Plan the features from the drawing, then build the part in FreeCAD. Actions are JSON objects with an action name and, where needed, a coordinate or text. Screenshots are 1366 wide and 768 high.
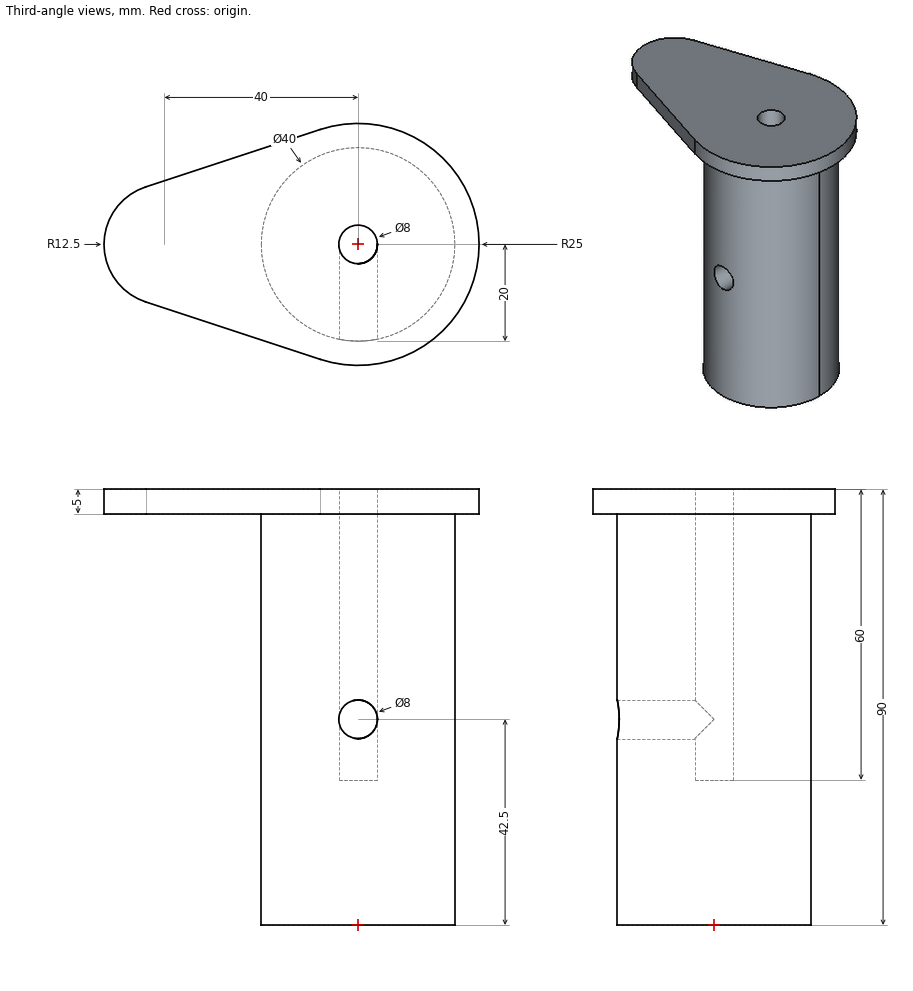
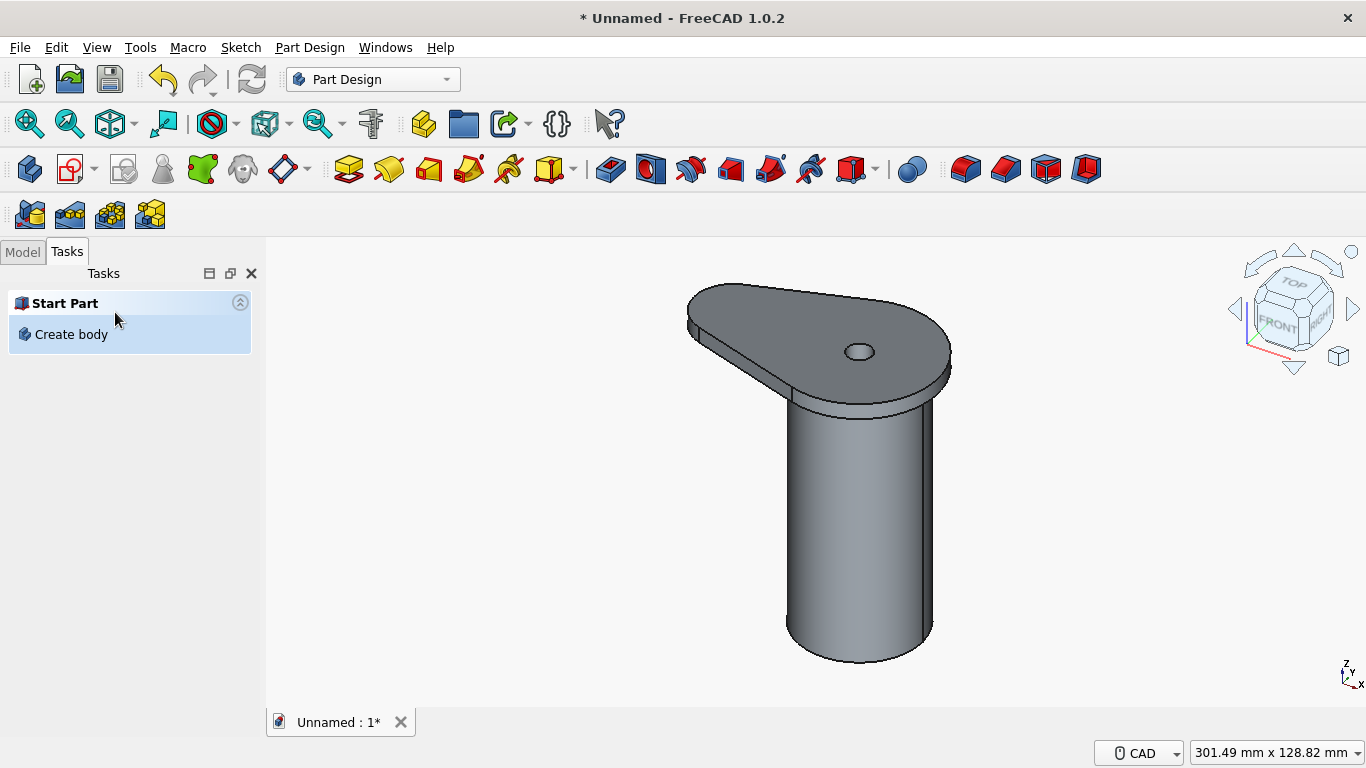
{"action": "left_click", "coordinate": [70, 170]}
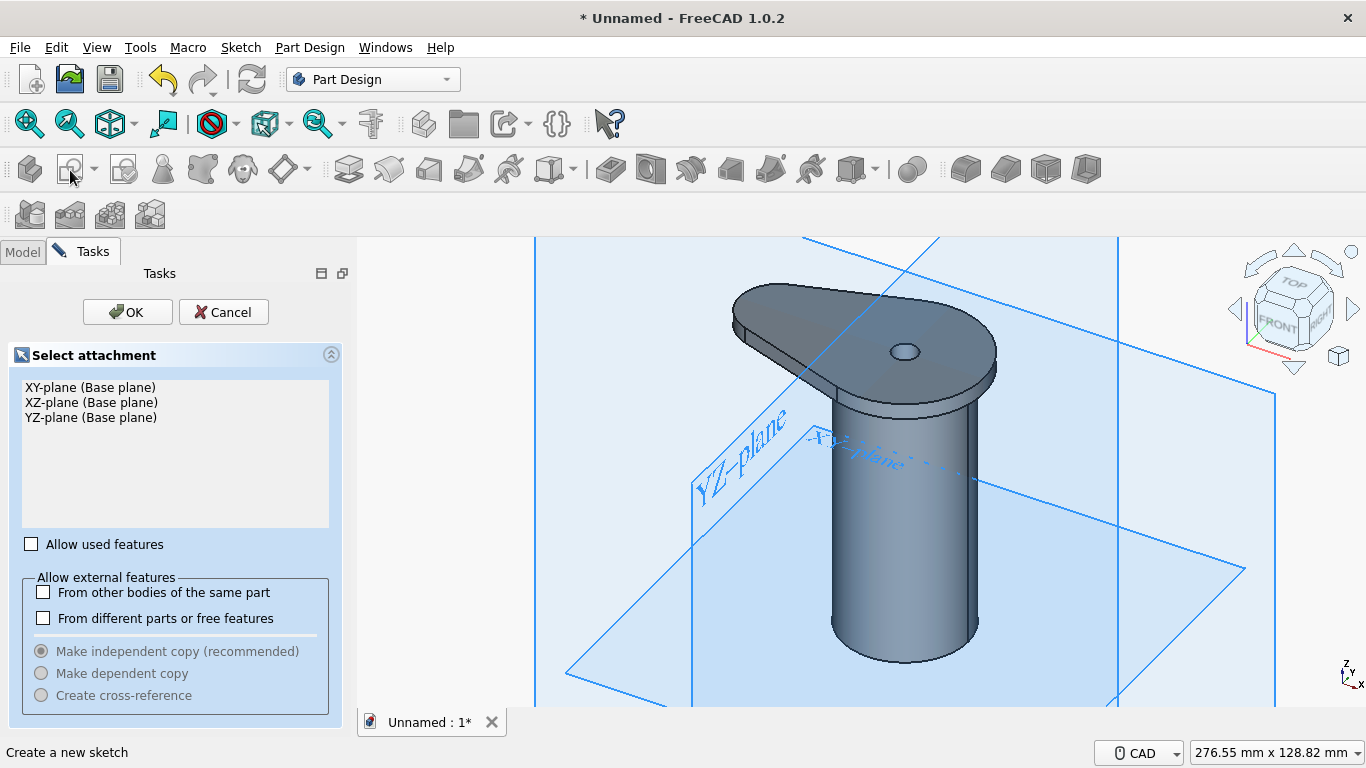
{"action": "left_click", "coordinate": [82, 402]}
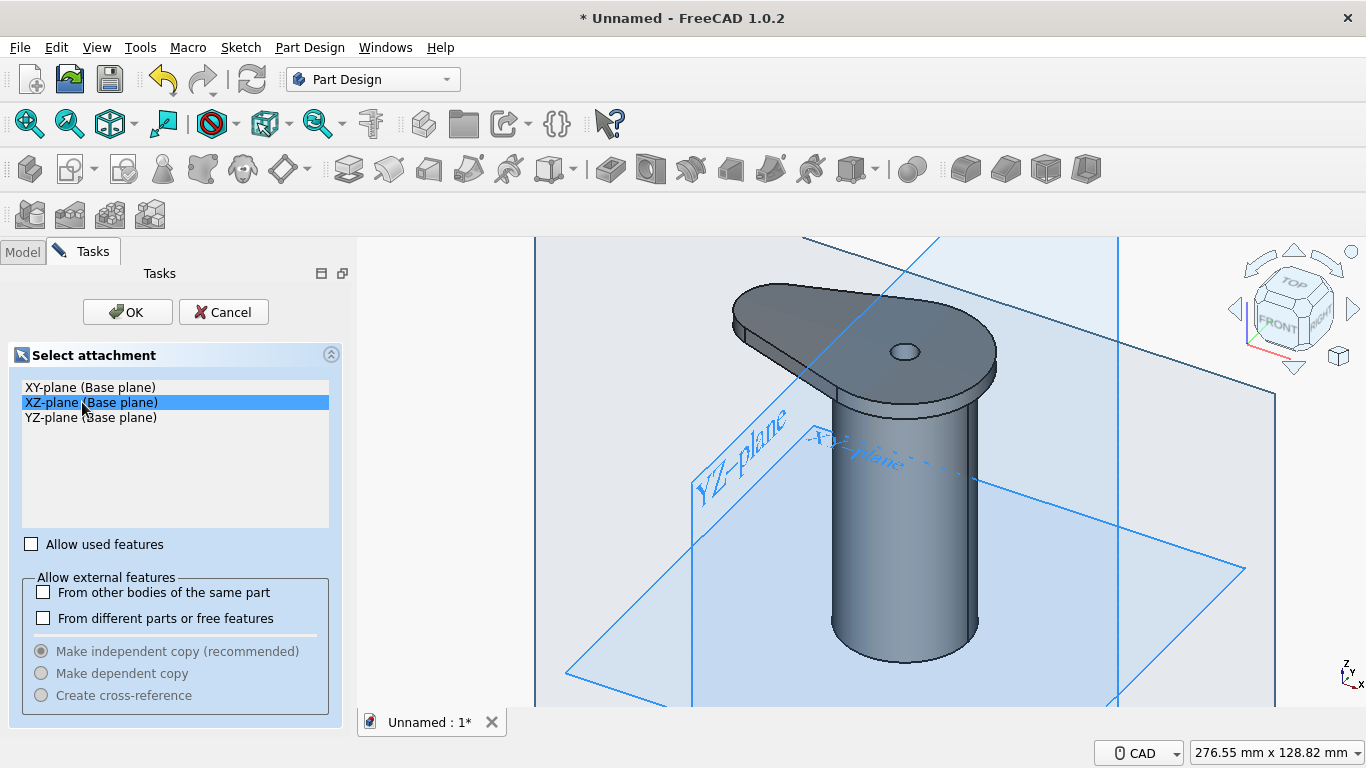
{"action": "left_click", "coordinate": [128, 312]}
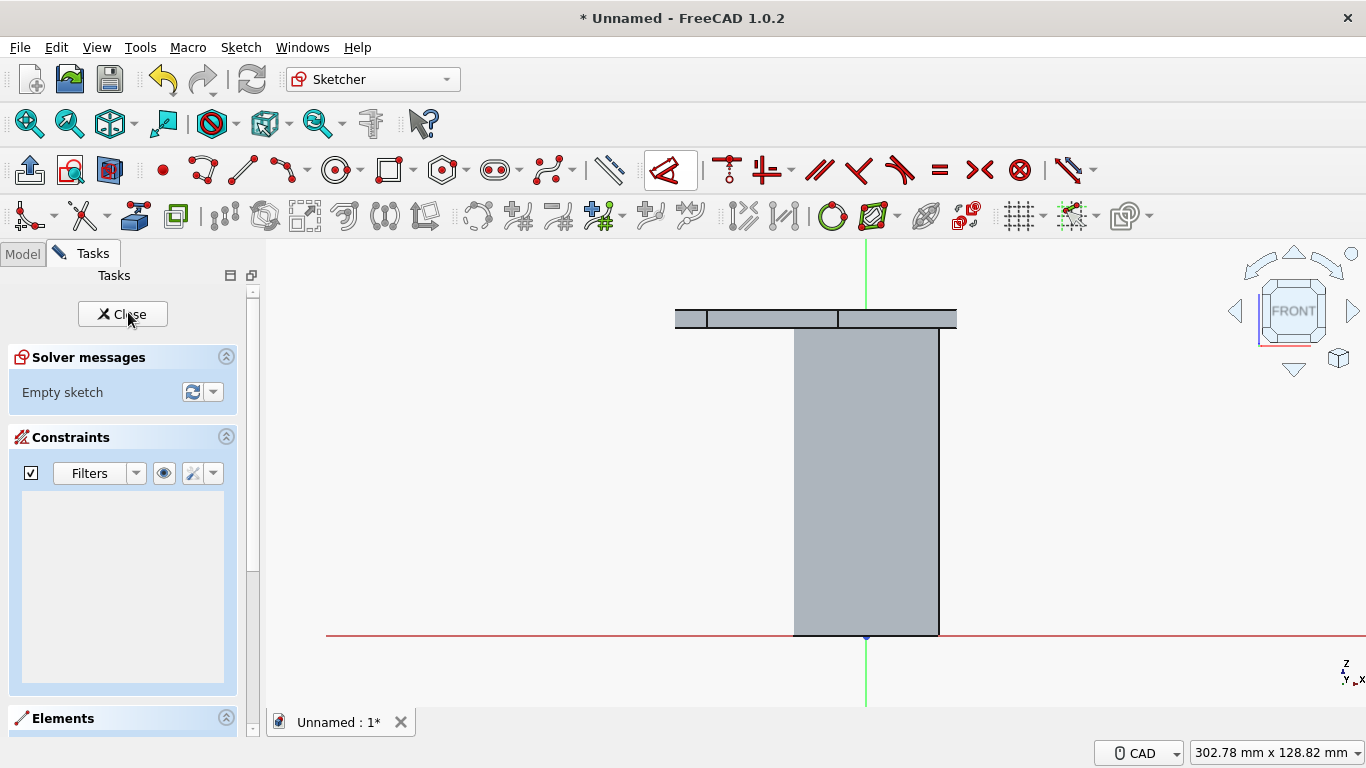
{"action": "left_click", "coordinate": [110, 170]}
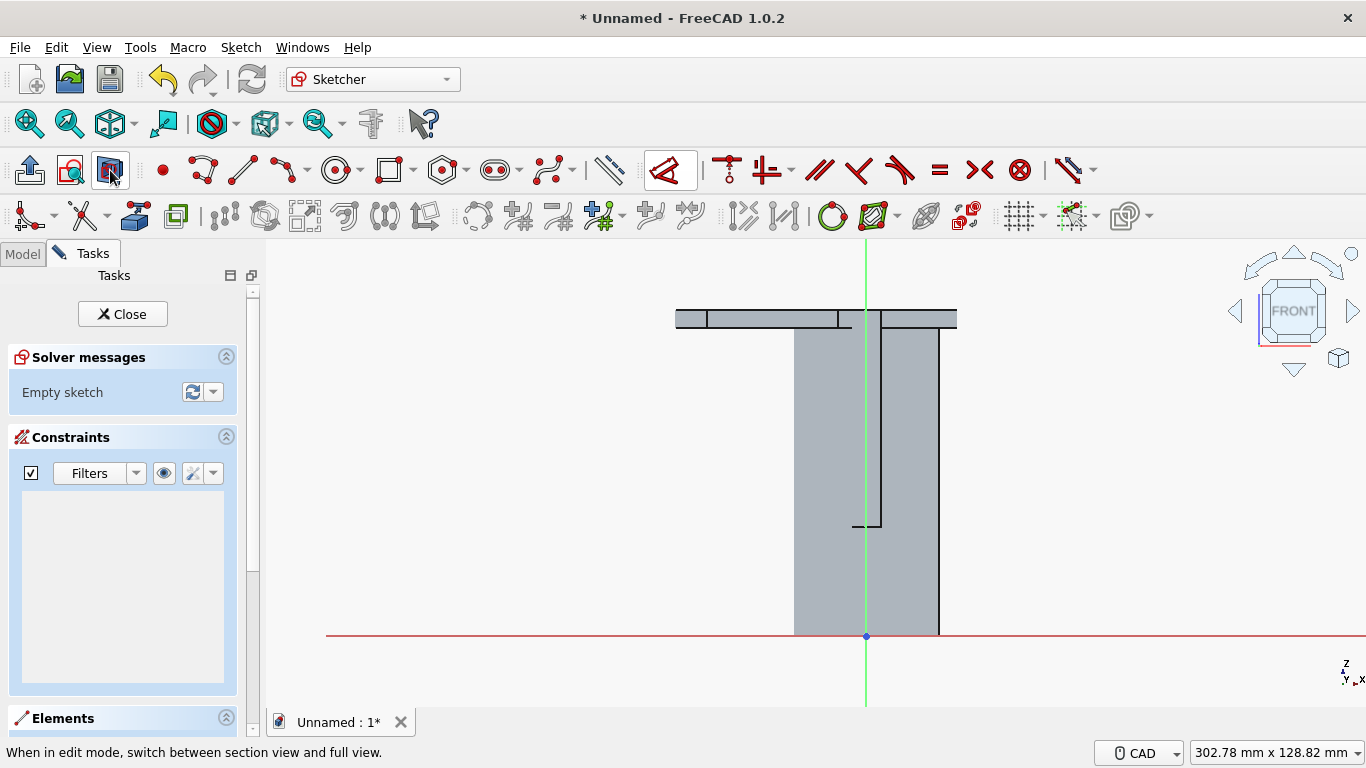
{"action": "scroll", "coordinate": [878, 483], "scroll_direction": "up", "scroll_amount": 12}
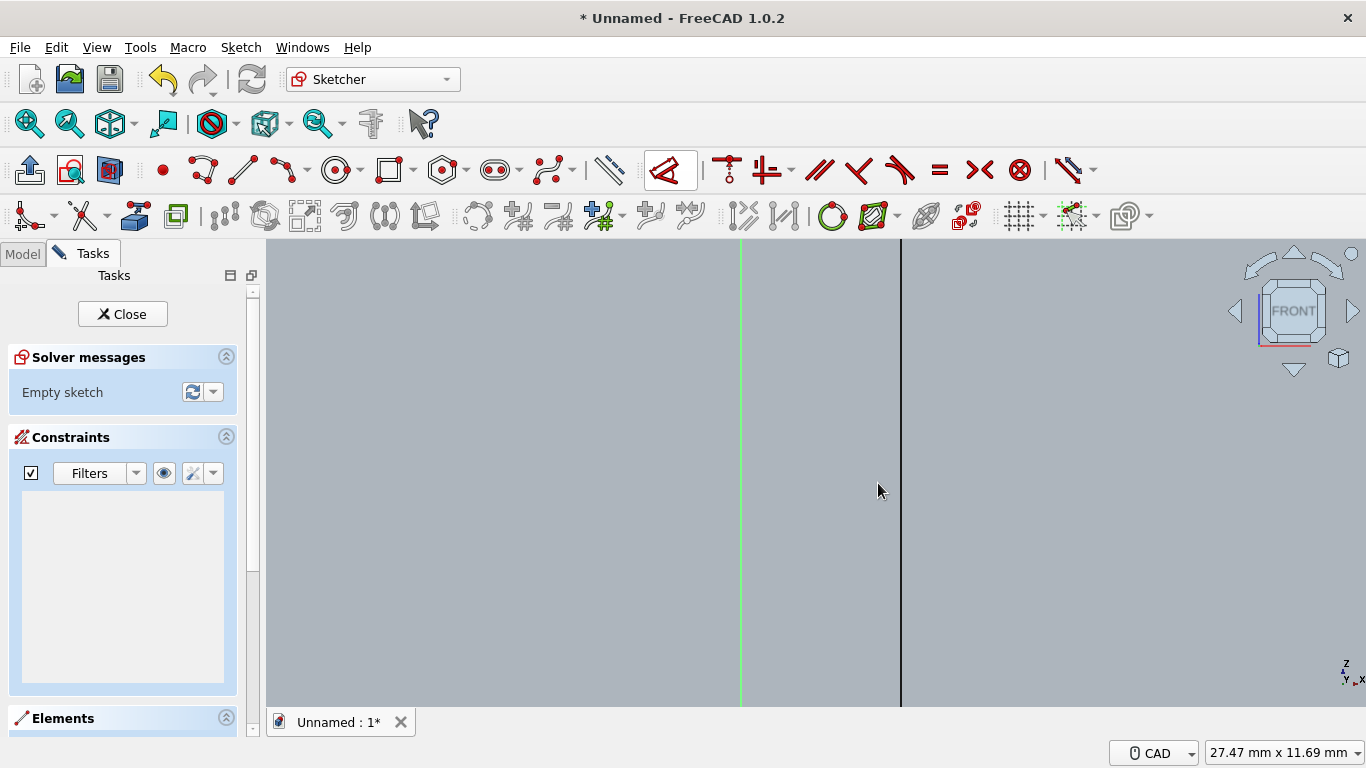
{"action": "key", "text": "g c"}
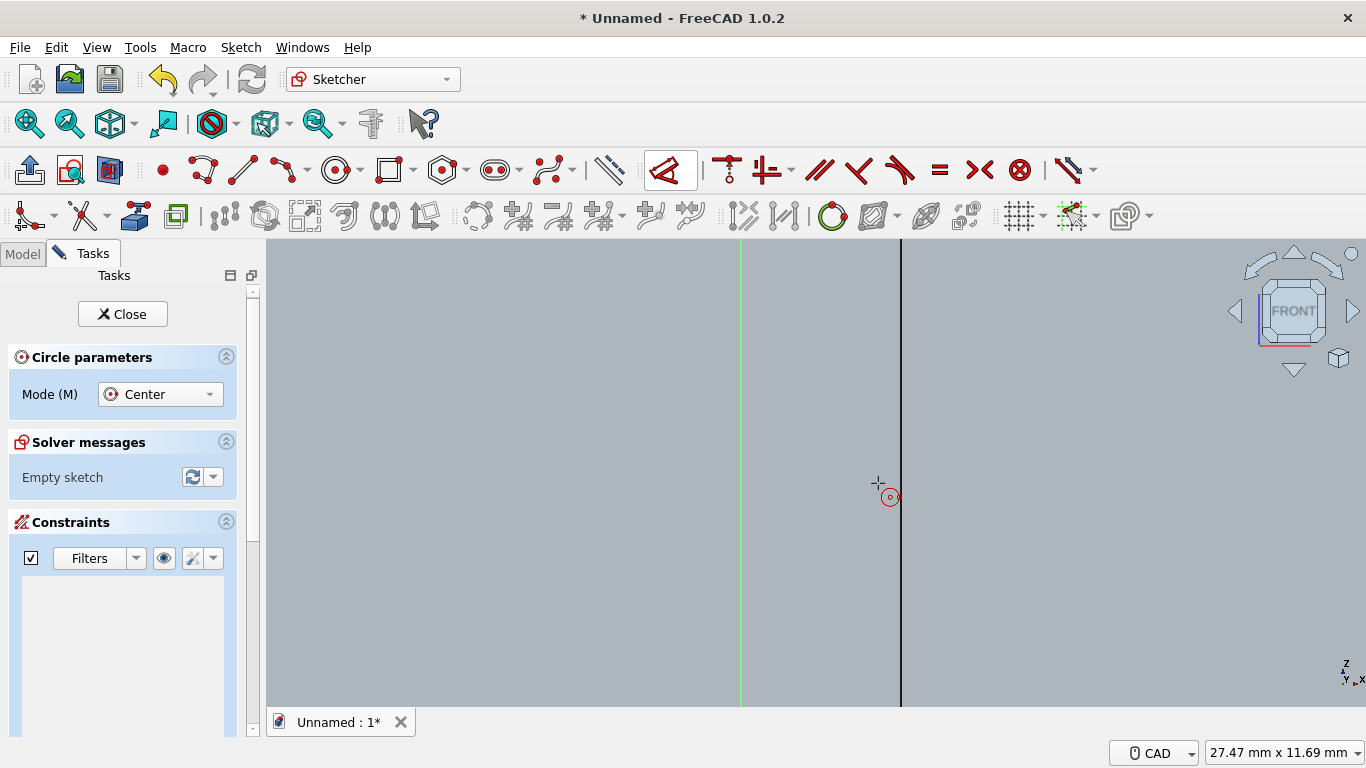
{"action": "left_click", "coordinate": [741, 468]}
{"action": "mouse_move", "coordinate": [854, 354]}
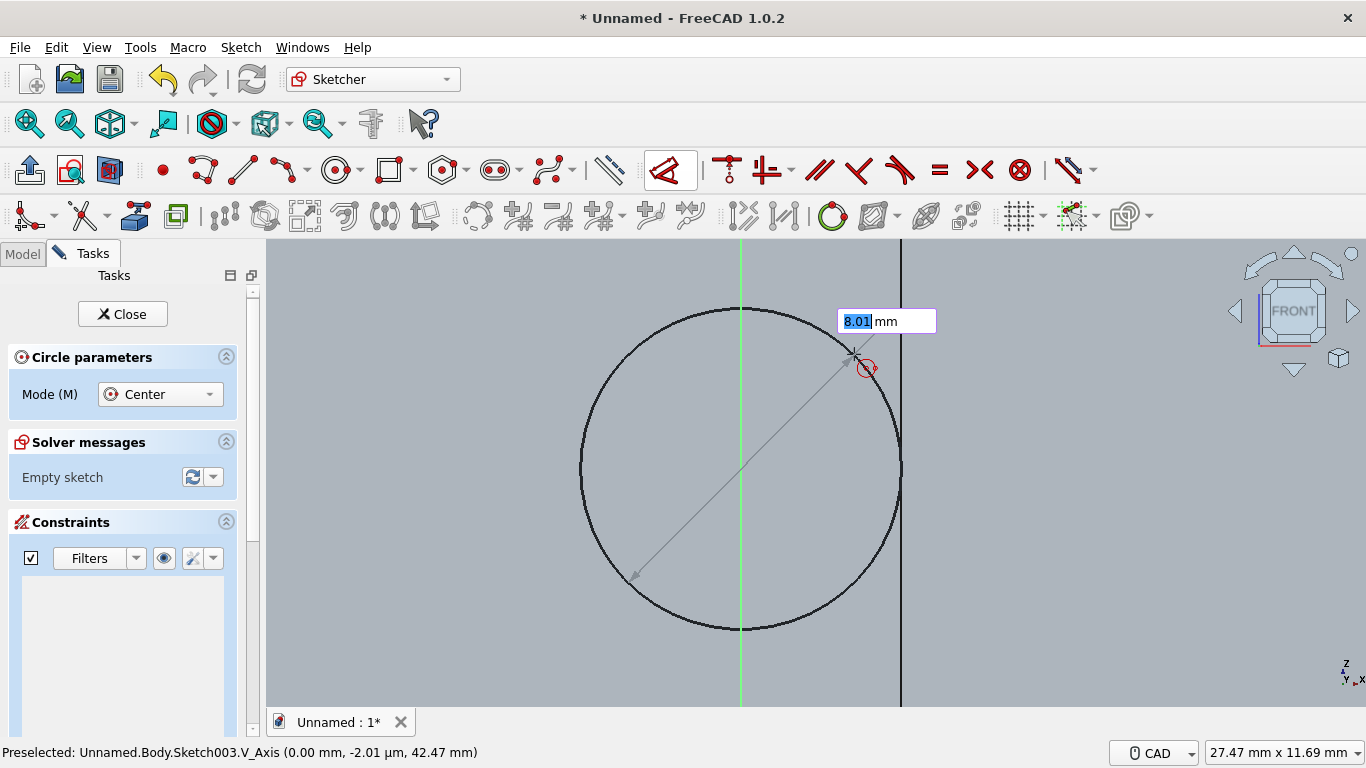
{"action": "type", "text": "8"}
{"action": "key", "text": "Return"}
{"action": "key", "text": "Escape"}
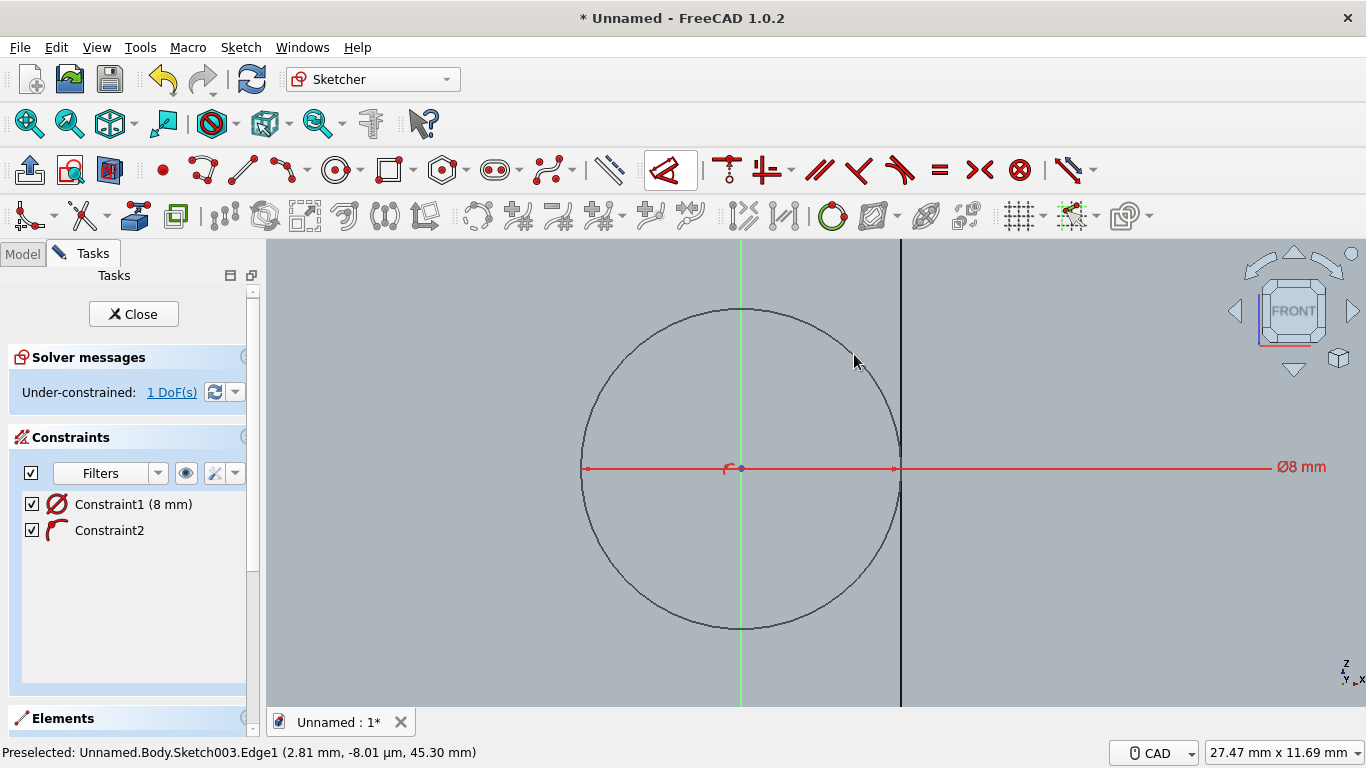
{"action": "left_click", "coordinate": [741, 469]}